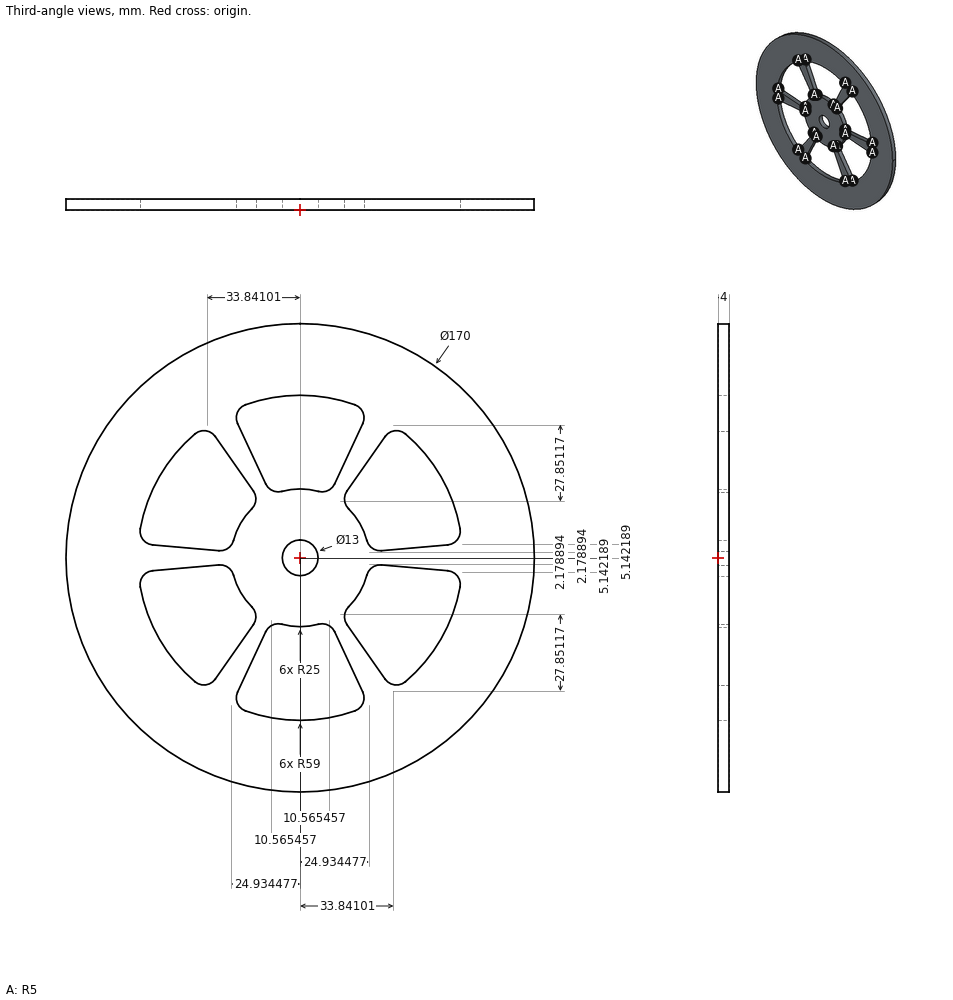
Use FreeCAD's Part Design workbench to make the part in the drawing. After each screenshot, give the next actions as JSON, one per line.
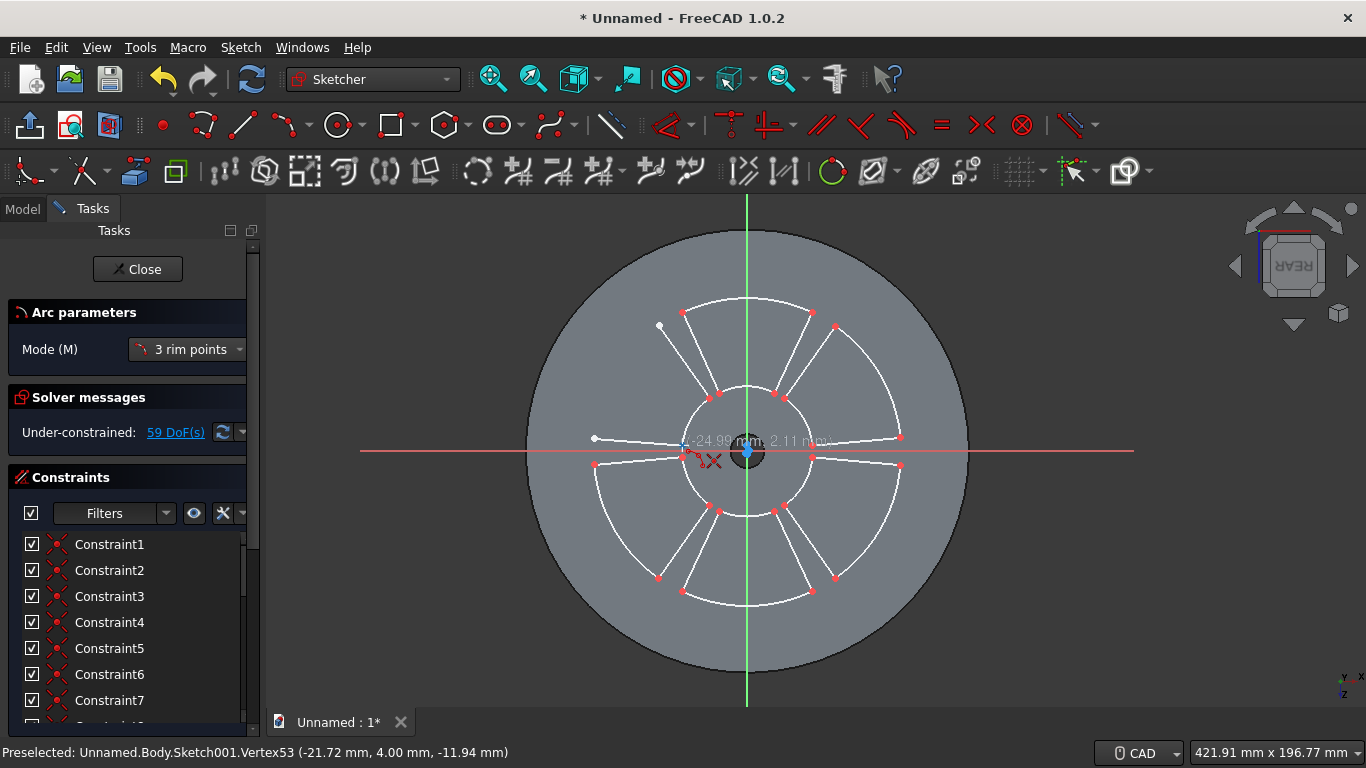
{"action": "left_click", "coordinate": [659, 326]}
{"action": "left_click", "coordinate": [594, 439]}
{"action": "left_click", "coordinate": [614, 374]}
{"action": "key", "text": "Escape"}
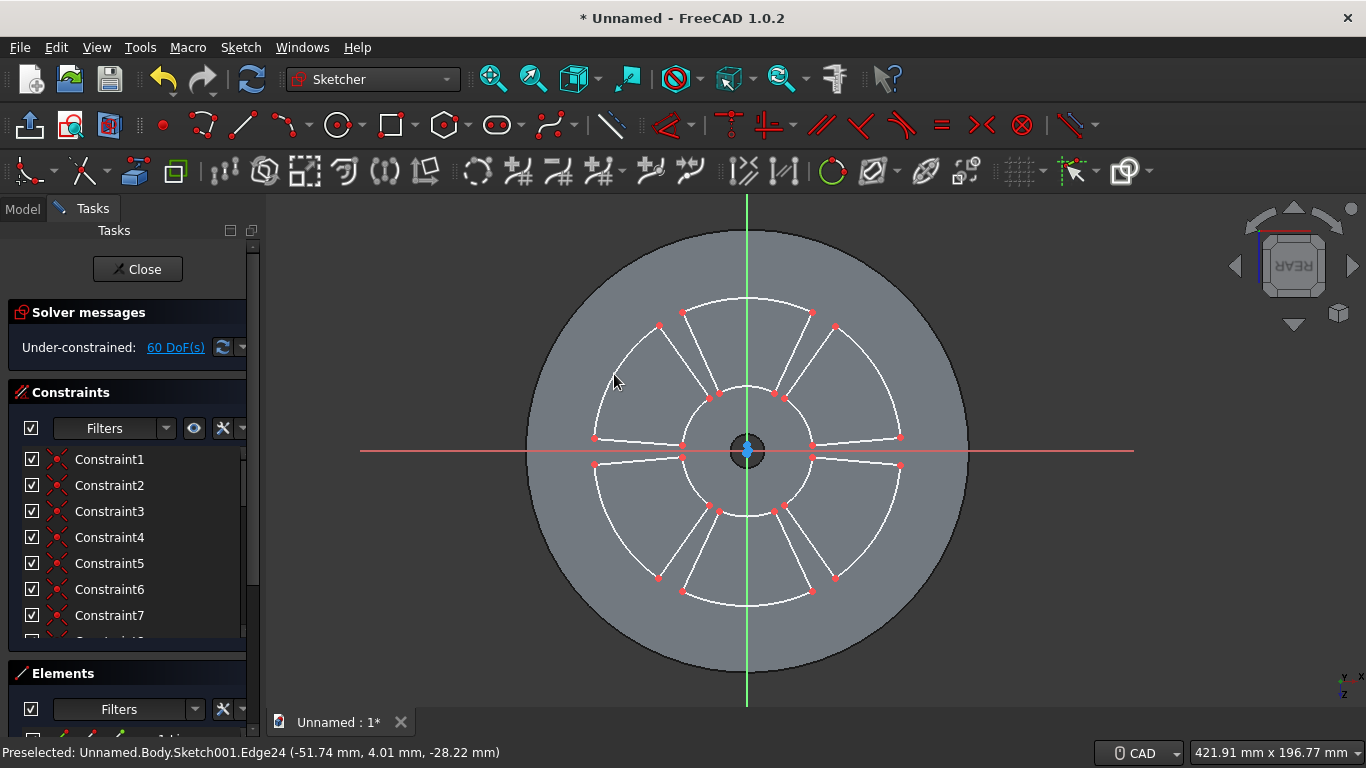
{"action": "left_click", "coordinate": [774, 300]}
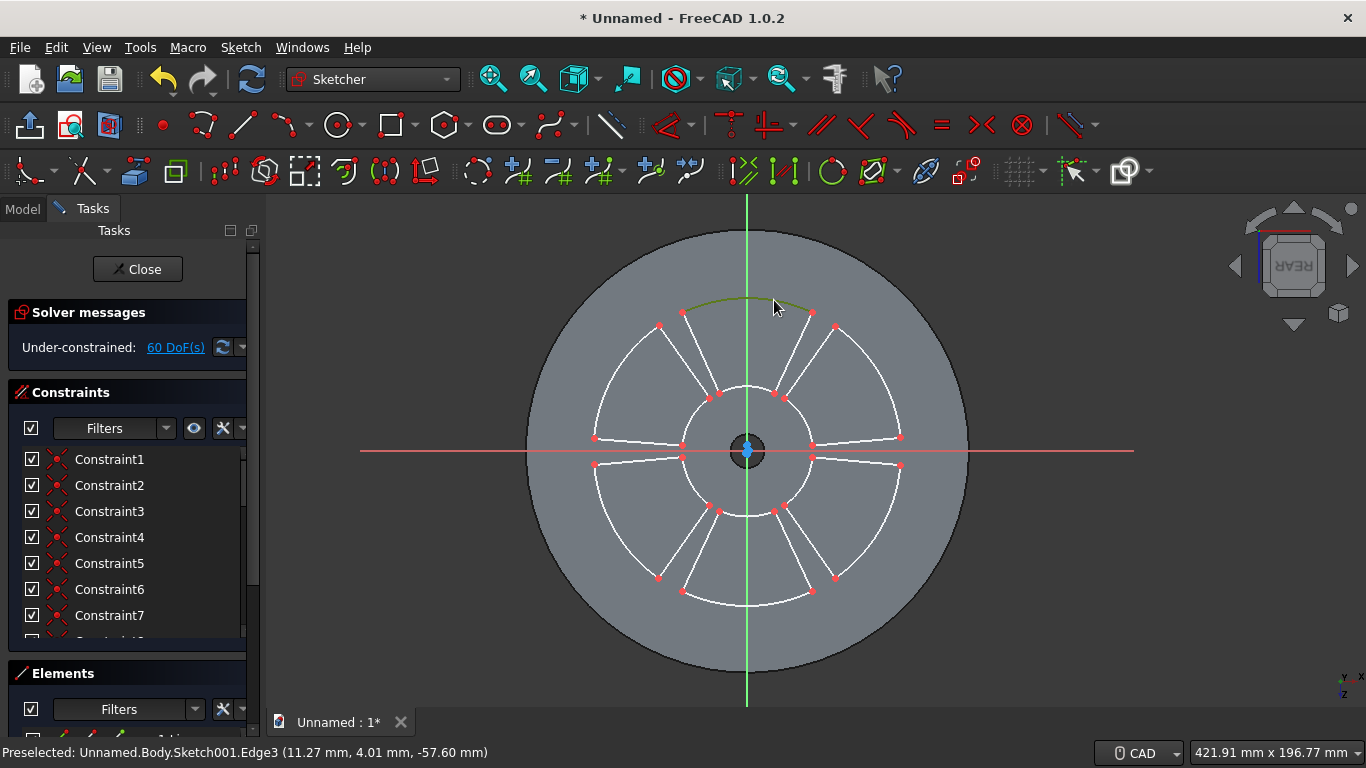
{"action": "scroll", "coordinate": [758, 387], "scroll_direction": "up", "scroll_amount": 2}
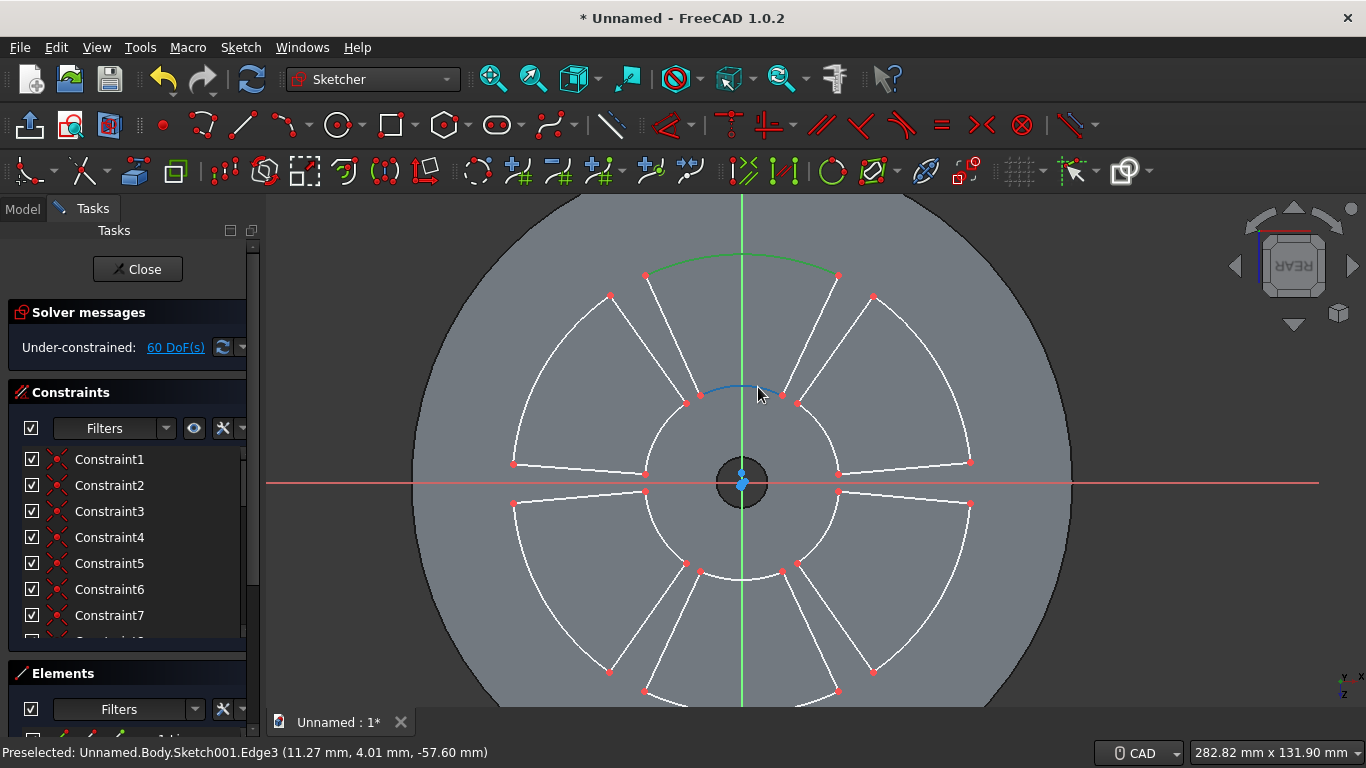
{"action": "left_click", "coordinate": [758, 387]}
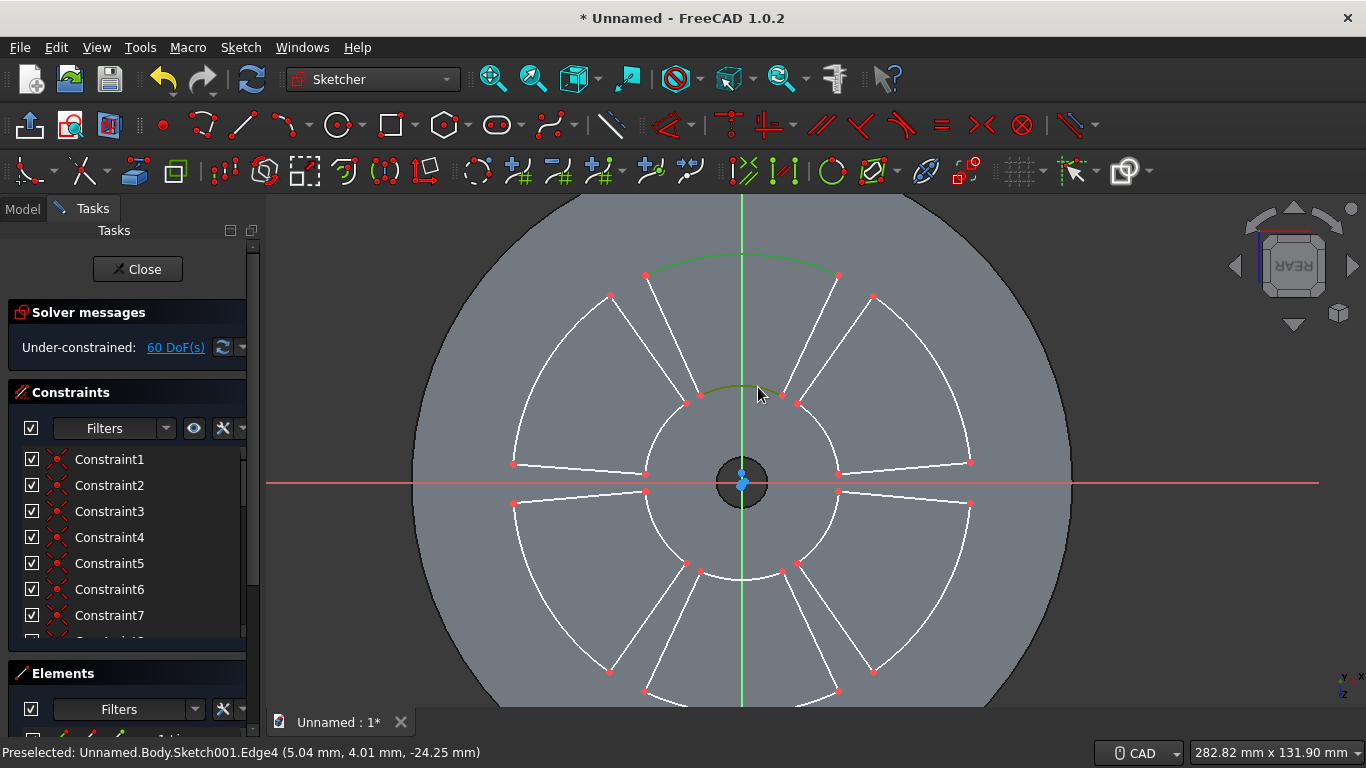
{"action": "left_click", "coordinate": [730, 126]}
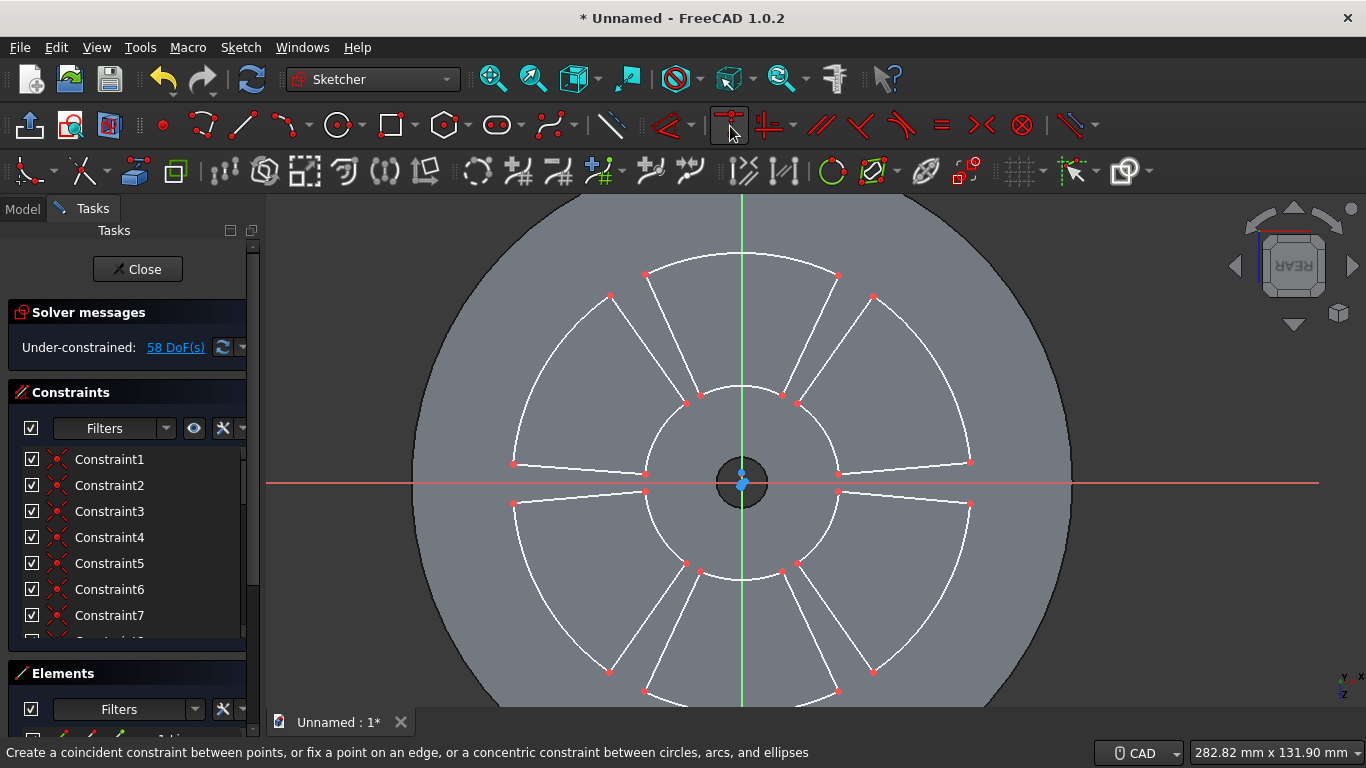
{"action": "left_click", "coordinate": [782, 257]}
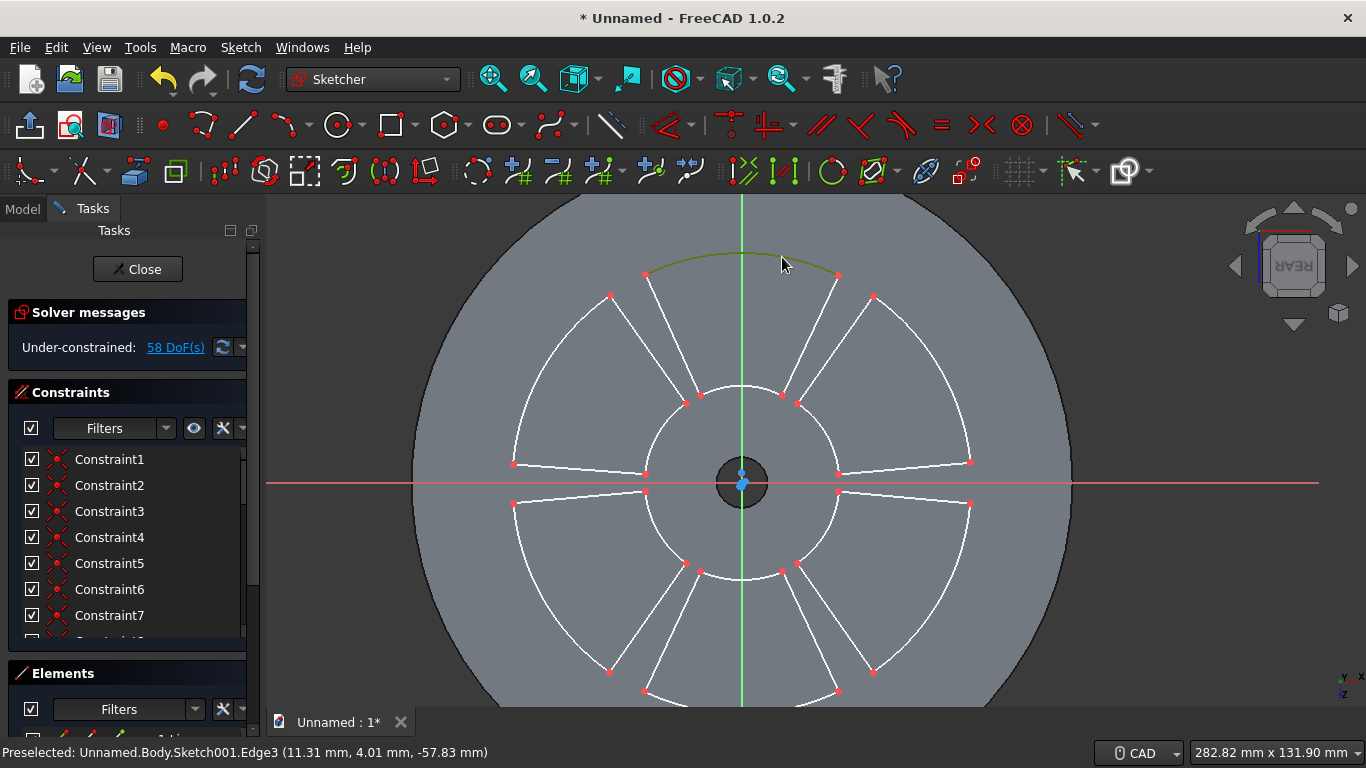
{"action": "left_click", "coordinate": [834, 450]}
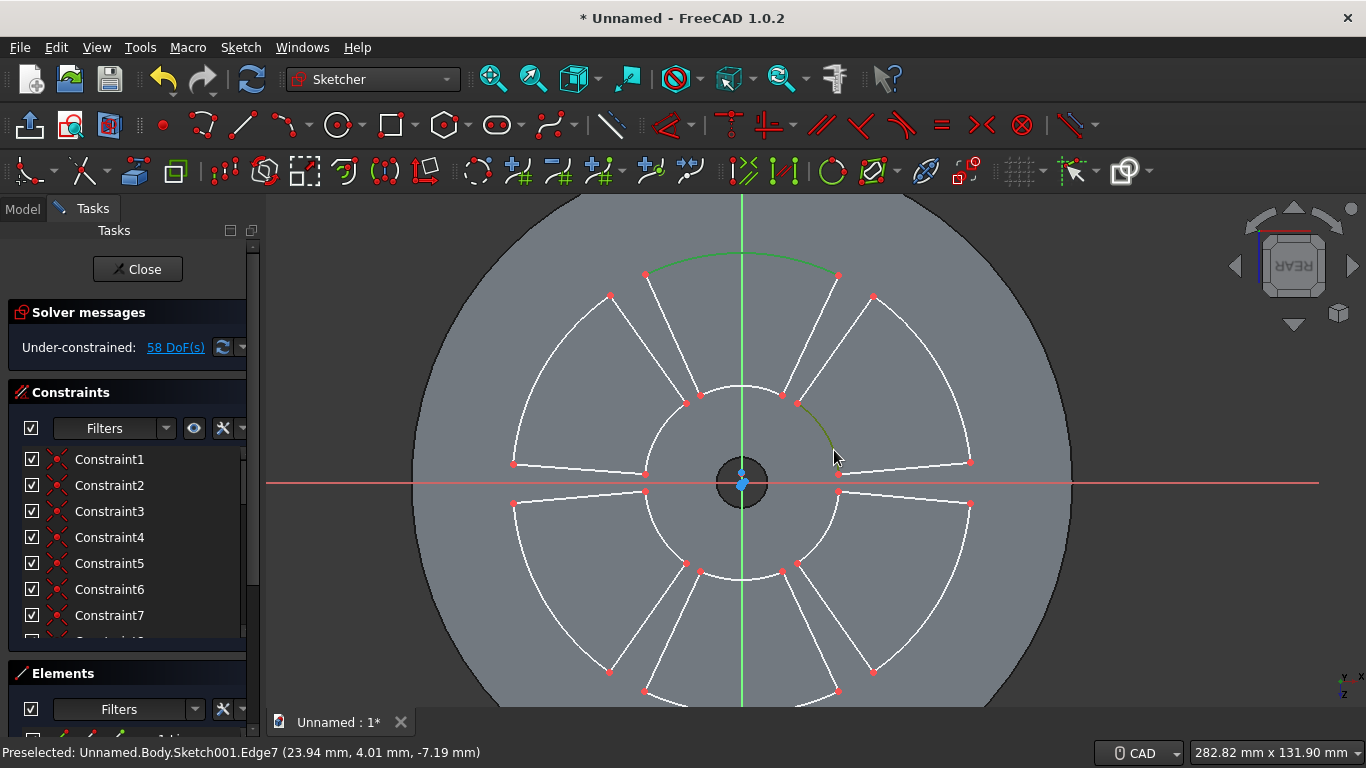
{"action": "left_click", "coordinate": [730, 126]}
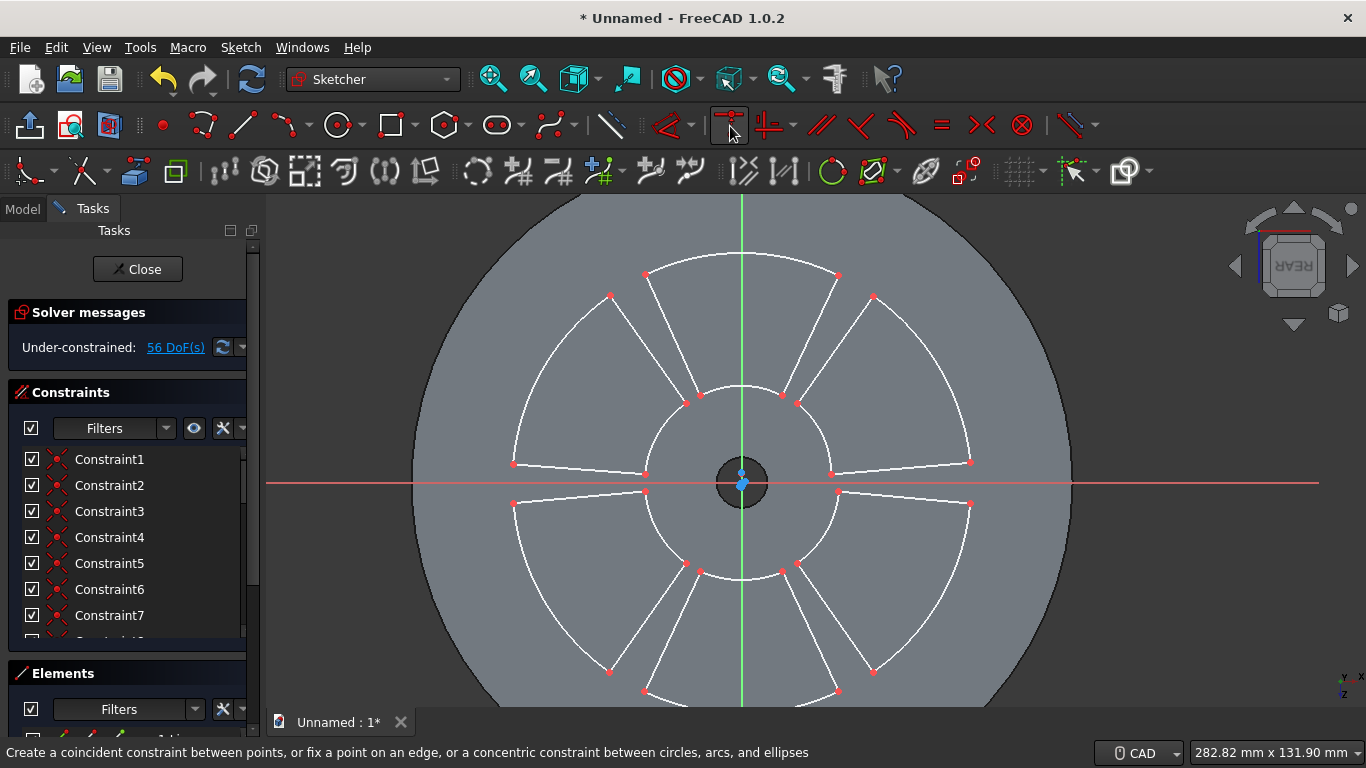
{"action": "left_click", "coordinate": [782, 257]}